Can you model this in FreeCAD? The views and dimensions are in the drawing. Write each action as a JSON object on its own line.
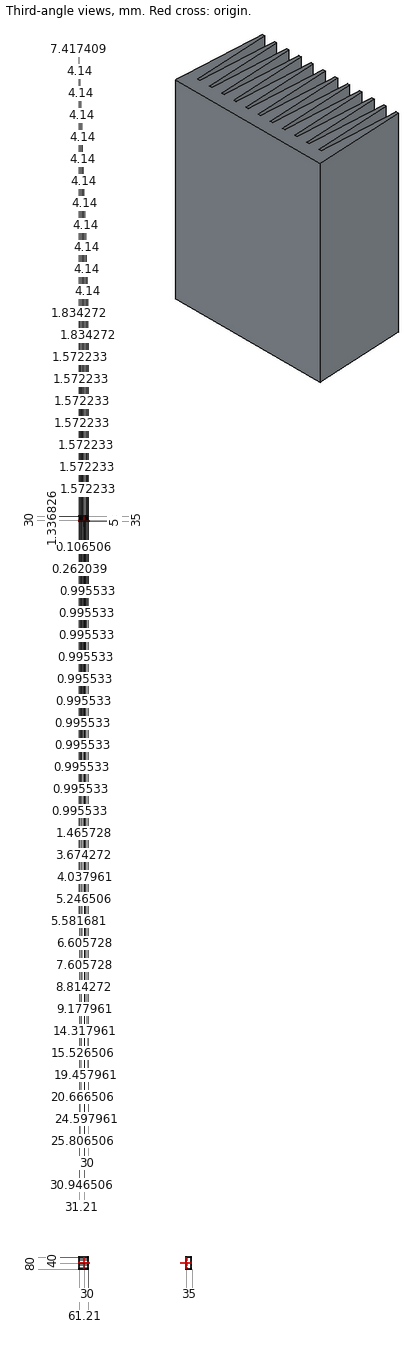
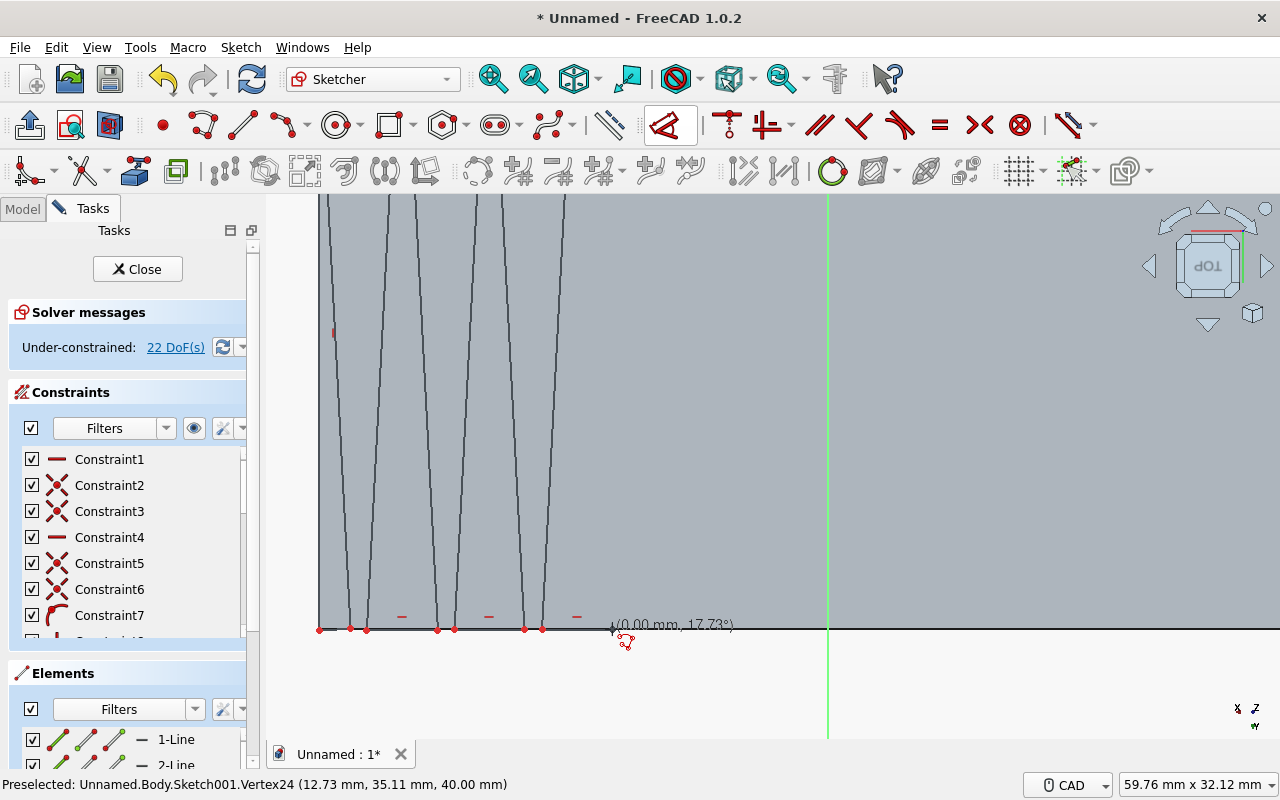
{"action": "scroll", "coordinate": [542, 630], "scroll_direction": "down", "scroll_amount": 3}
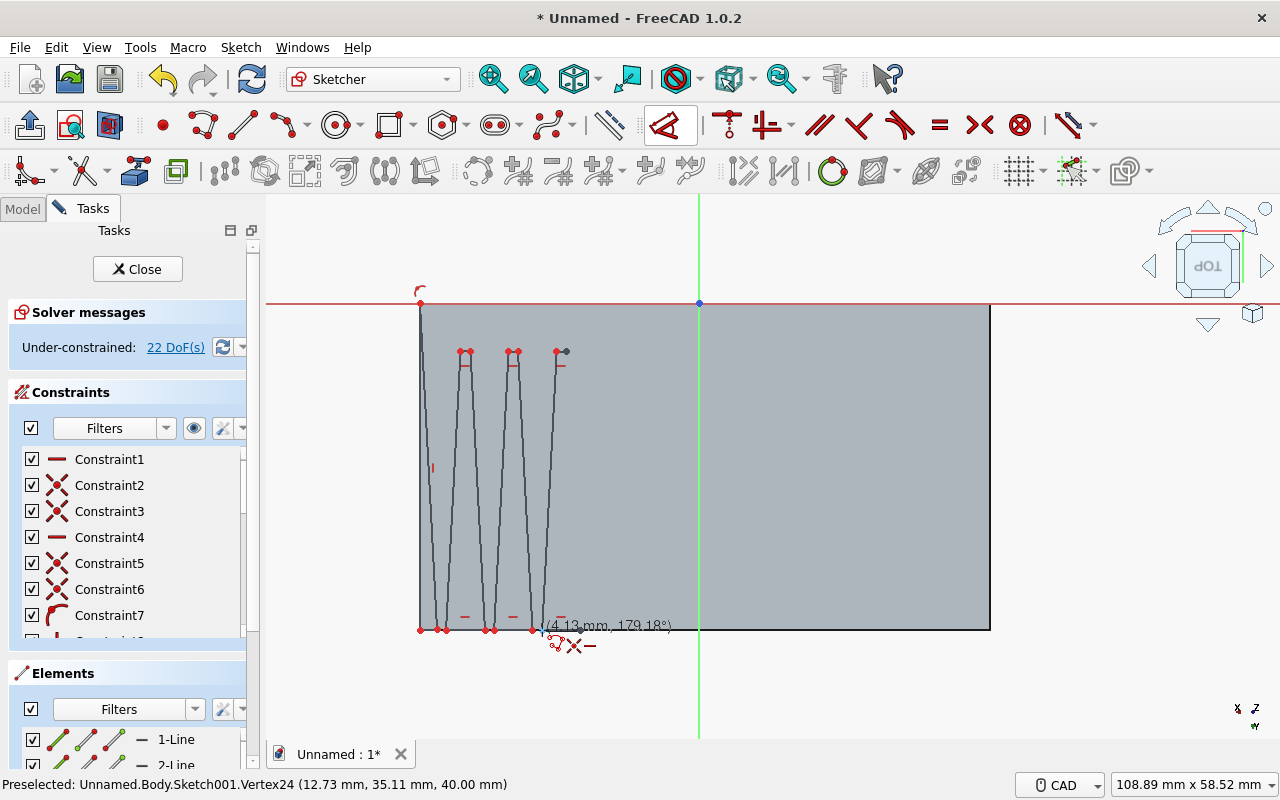
{"action": "scroll", "coordinate": [566, 351], "scroll_direction": "up", "scroll_amount": 7}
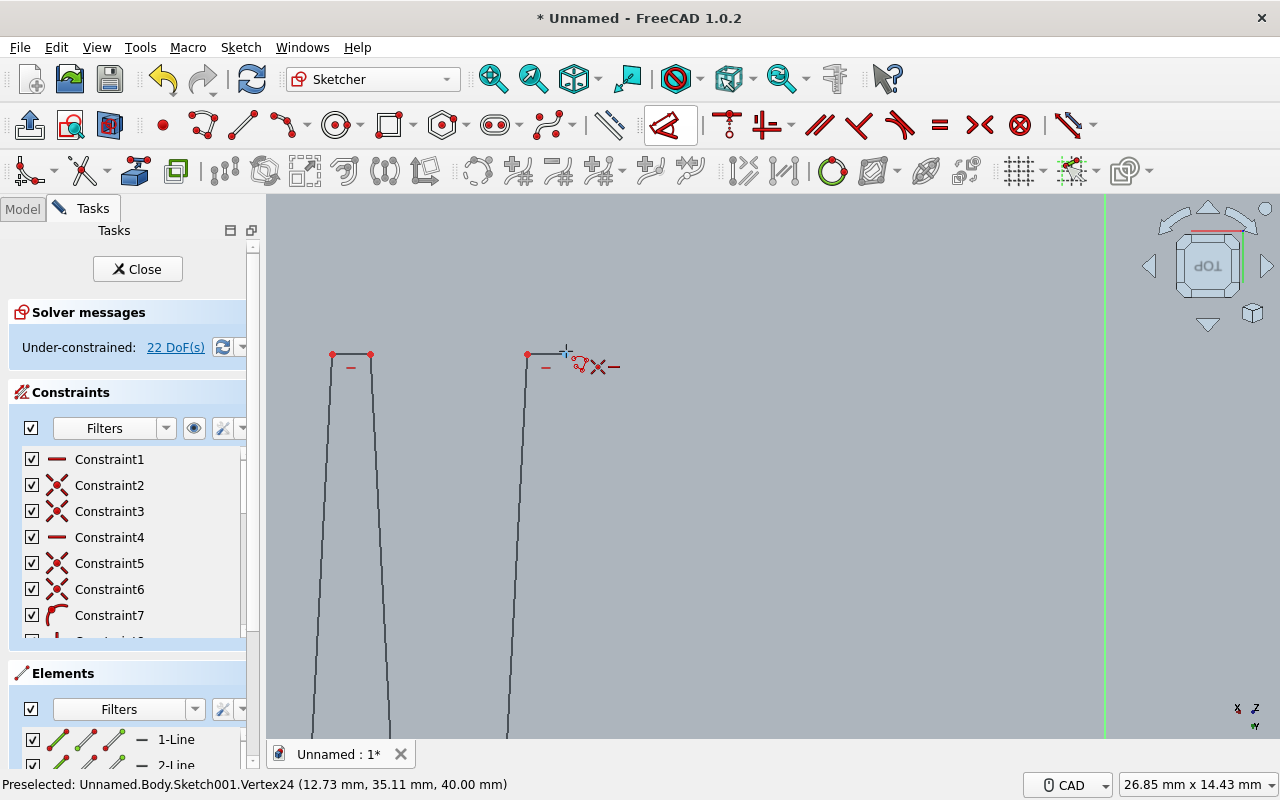
{"action": "left_click", "coordinate": [565, 354]}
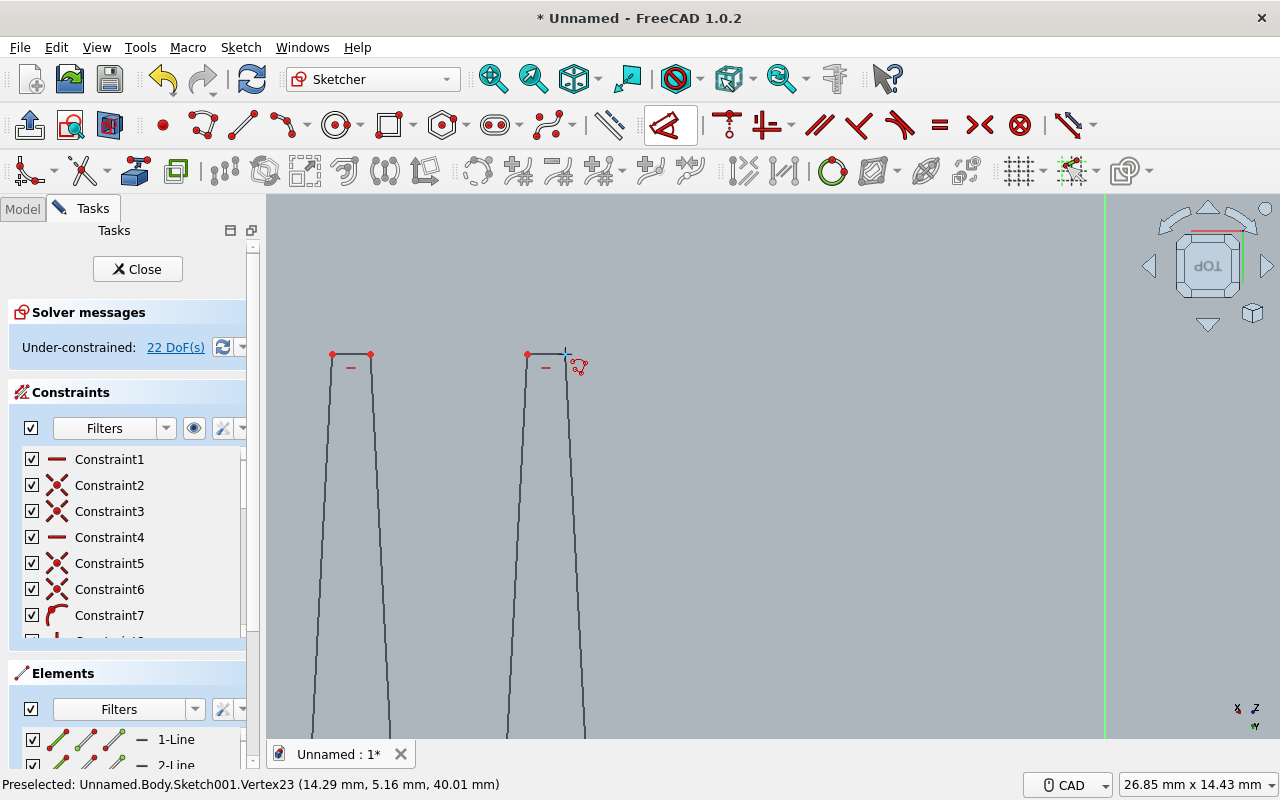
{"action": "scroll", "coordinate": [566, 351], "scroll_direction": "down", "scroll_amount": 7}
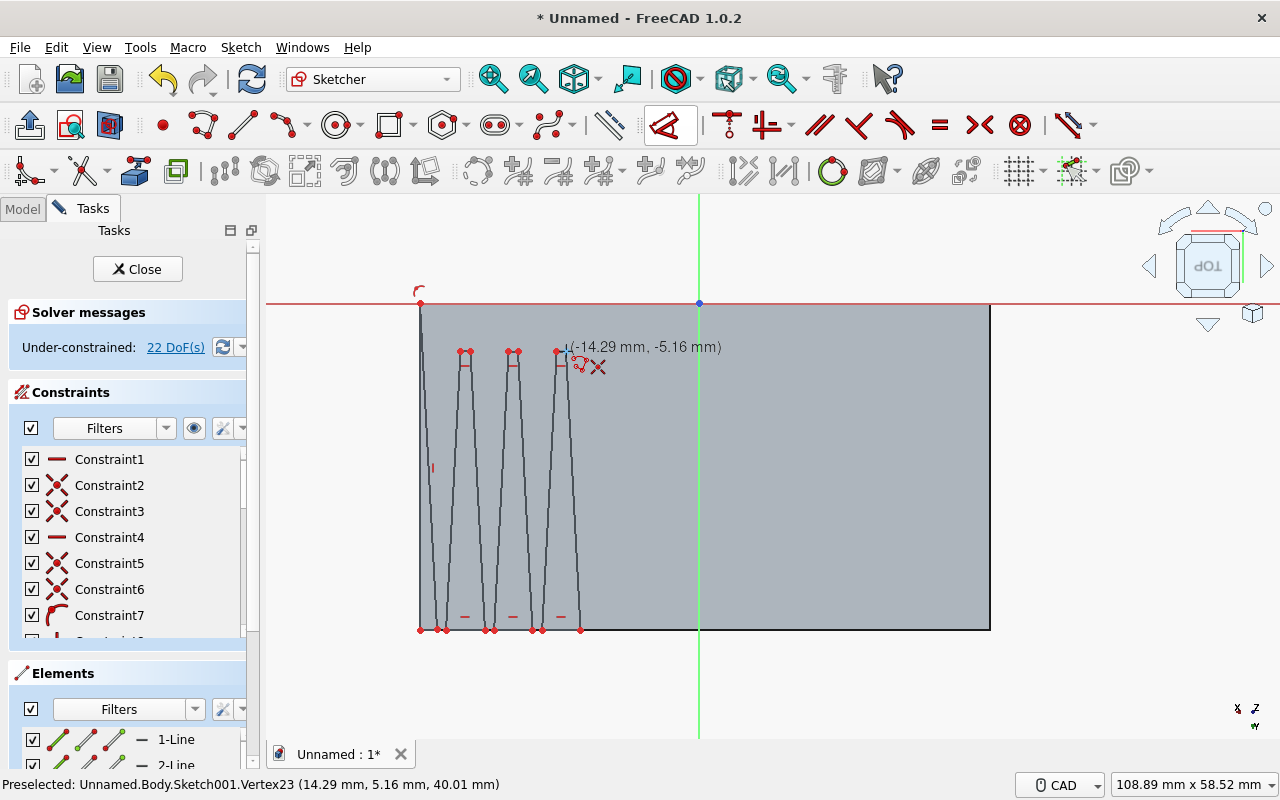
{"action": "left_click", "coordinate": [614, 351]}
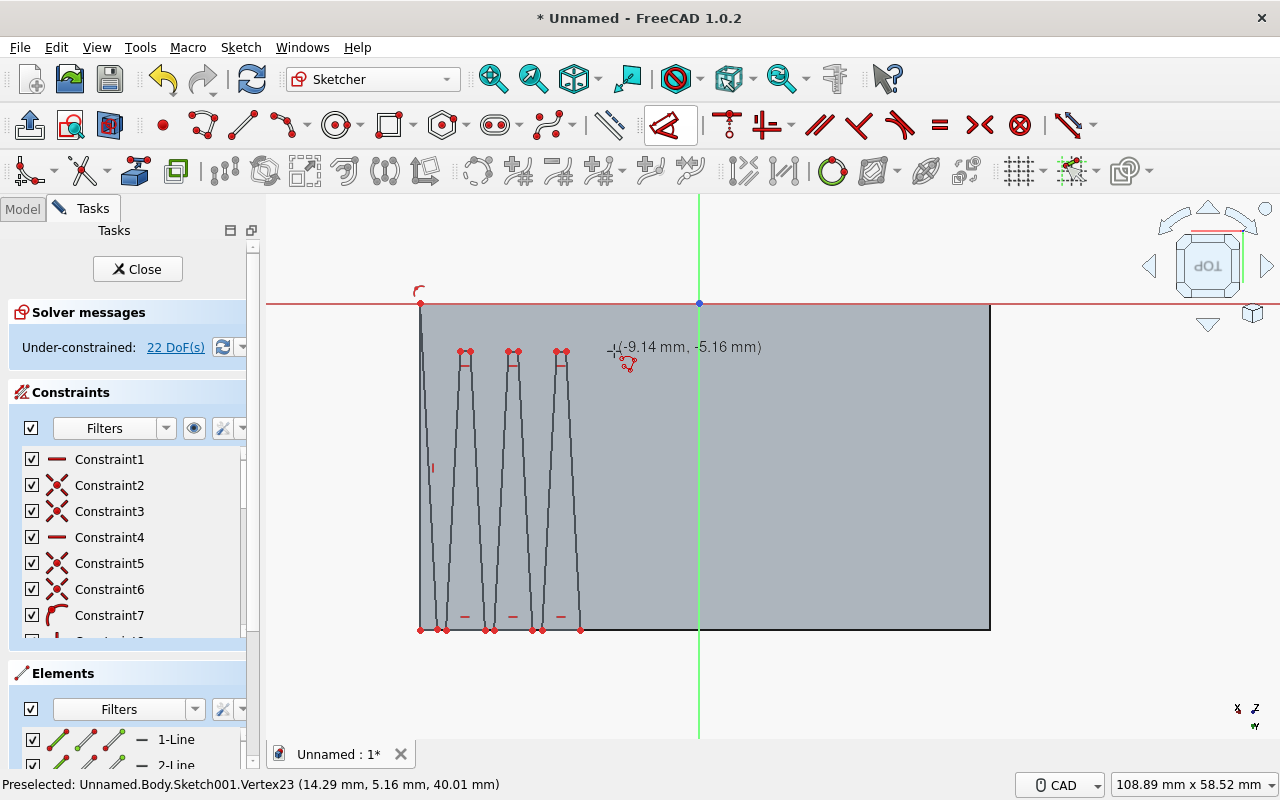
{"action": "scroll", "coordinate": [604, 351], "scroll_direction": "up", "scroll_amount": 3}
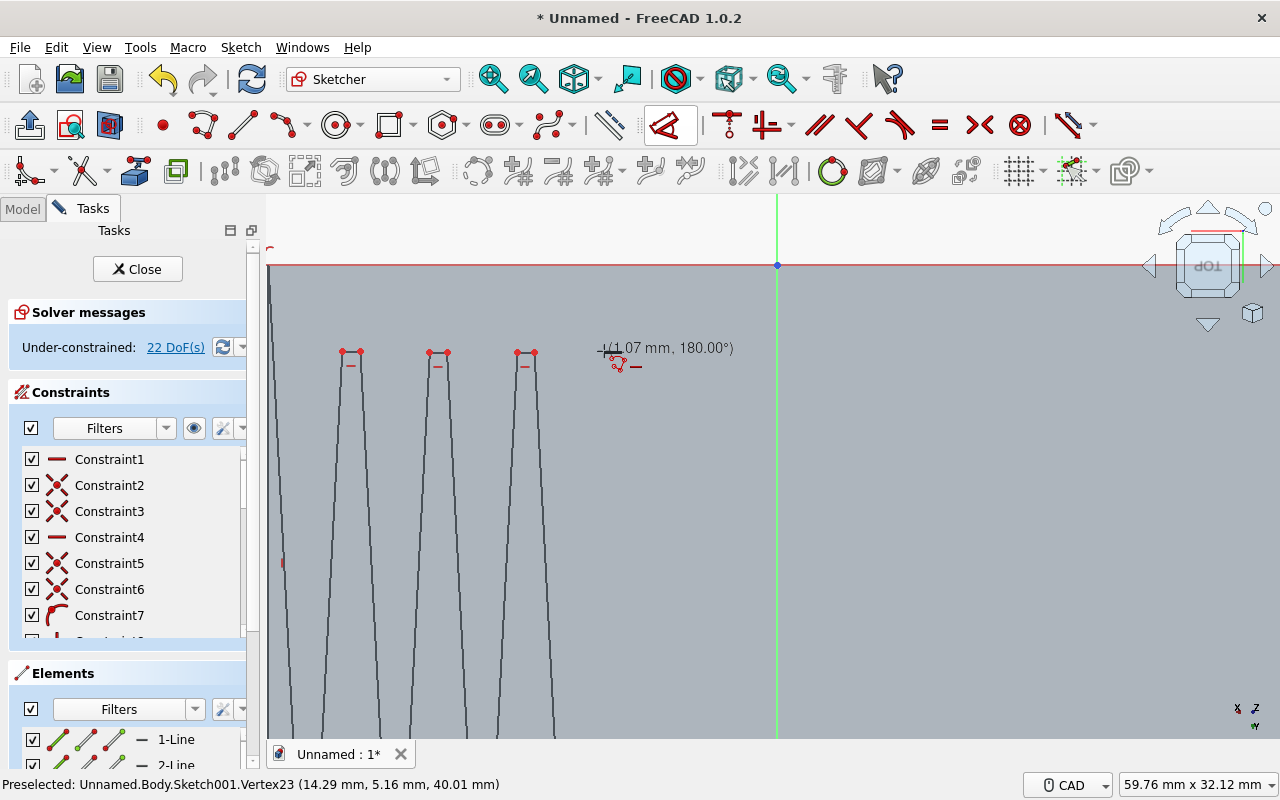
{"action": "left_click", "coordinate": [604, 351]}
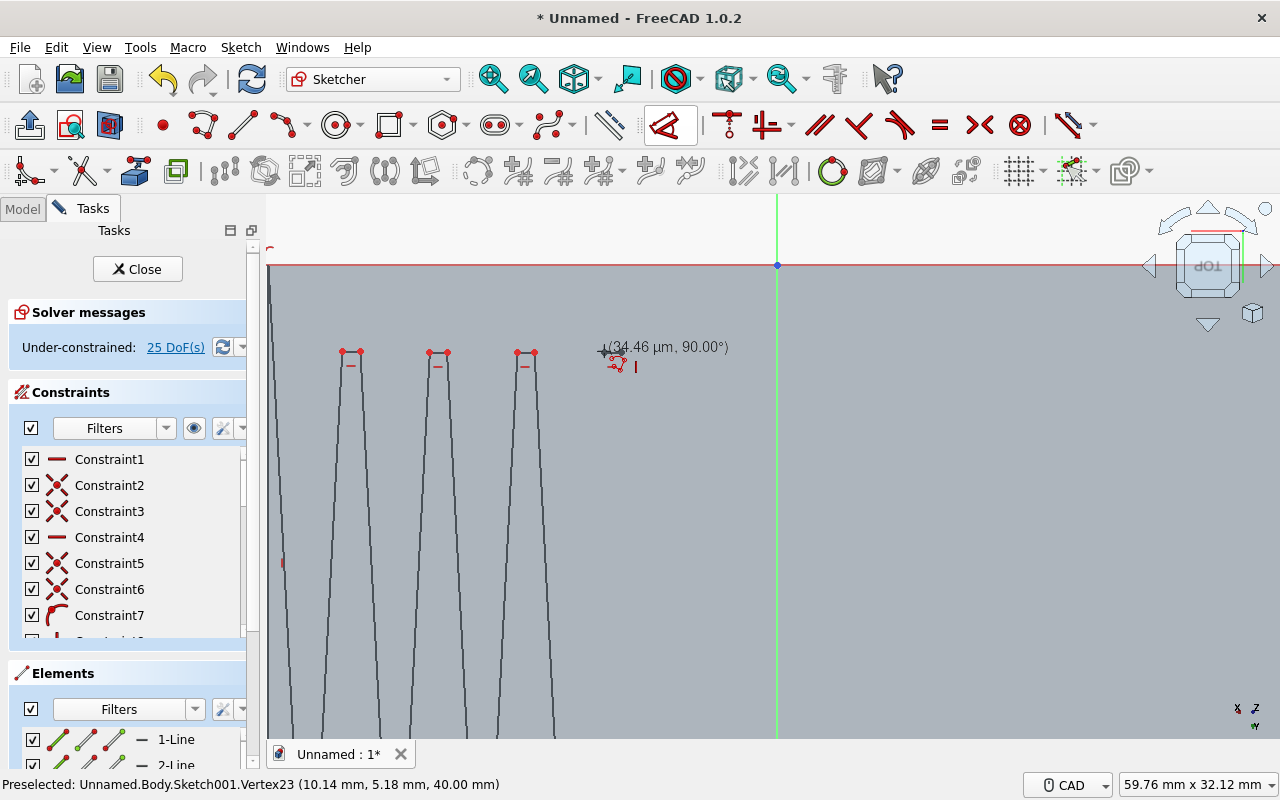
{"action": "scroll", "coordinate": [604, 350], "scroll_direction": "down", "scroll_amount": 3}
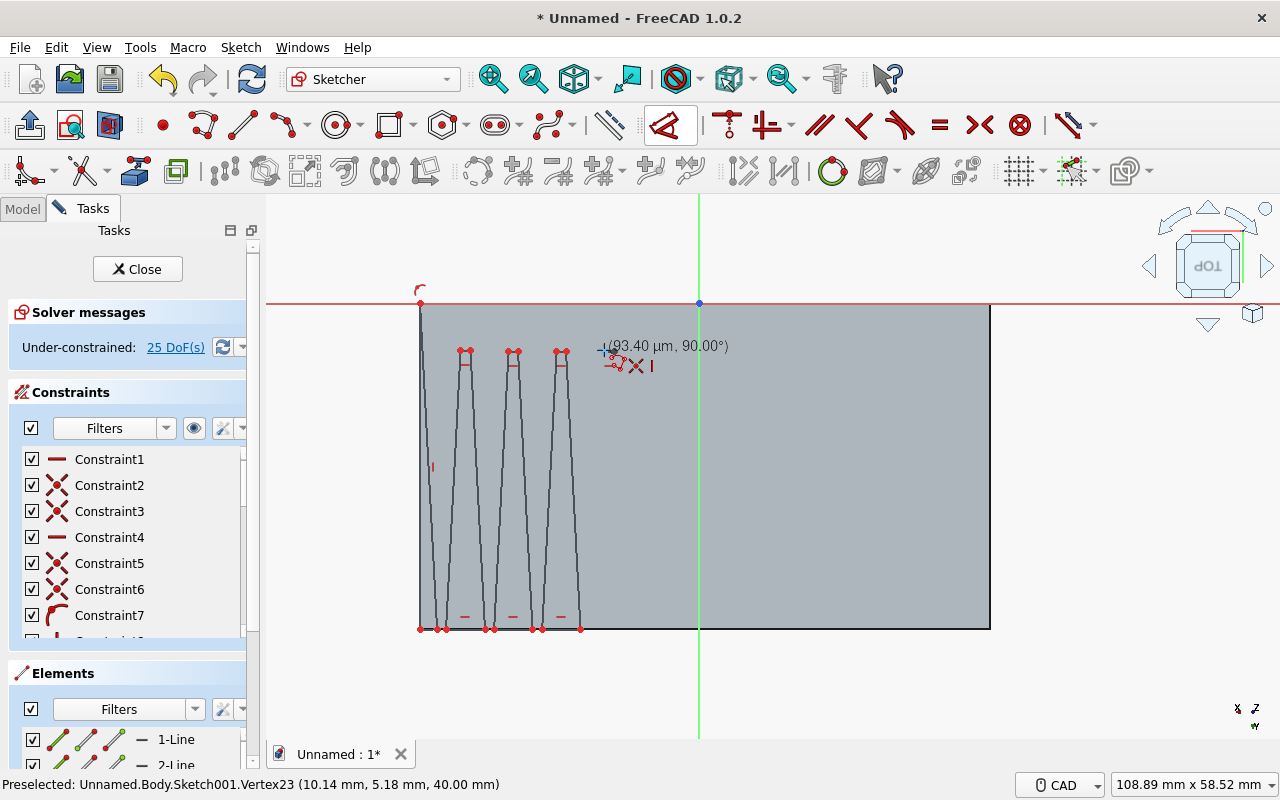
{"action": "scroll", "coordinate": [590, 629], "scroll_direction": "up", "scroll_amount": 3}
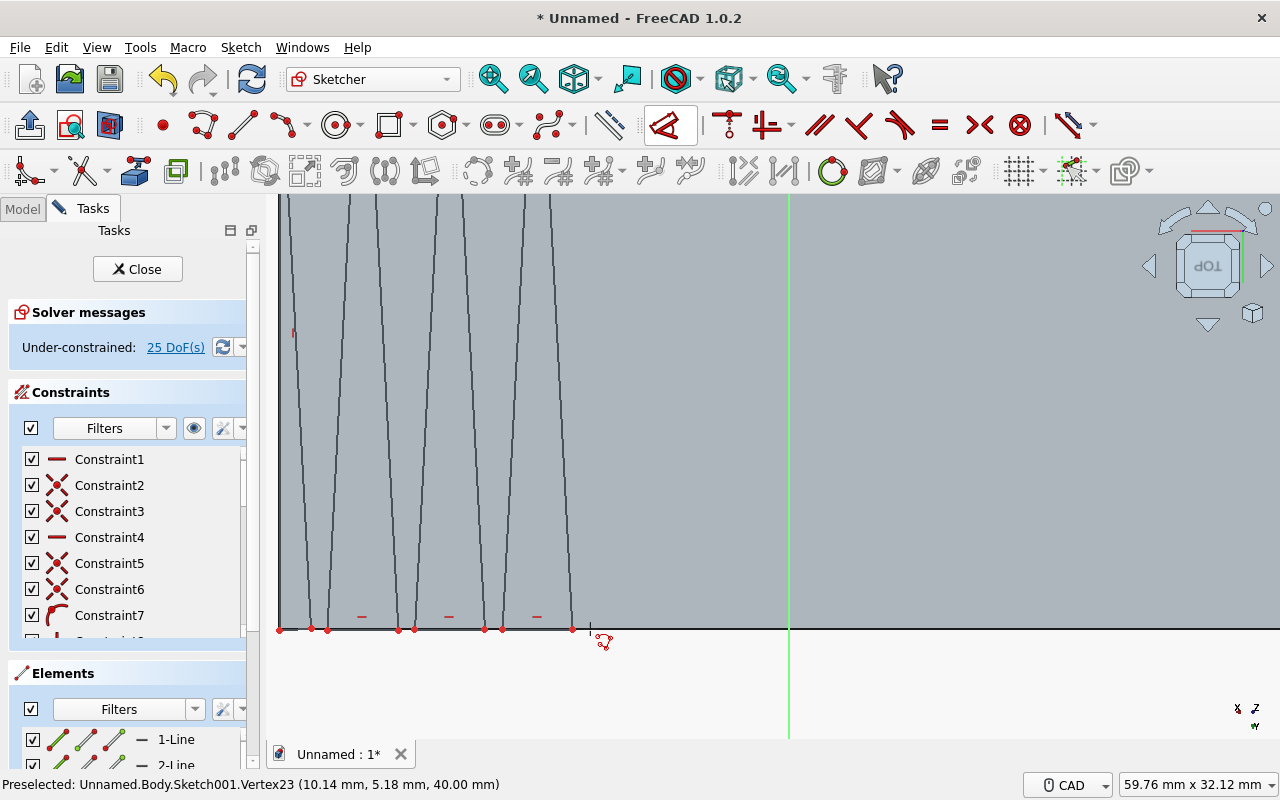
{"action": "left_click", "coordinate": [589, 629]}
{"action": "left_click", "coordinate": [659, 629]}